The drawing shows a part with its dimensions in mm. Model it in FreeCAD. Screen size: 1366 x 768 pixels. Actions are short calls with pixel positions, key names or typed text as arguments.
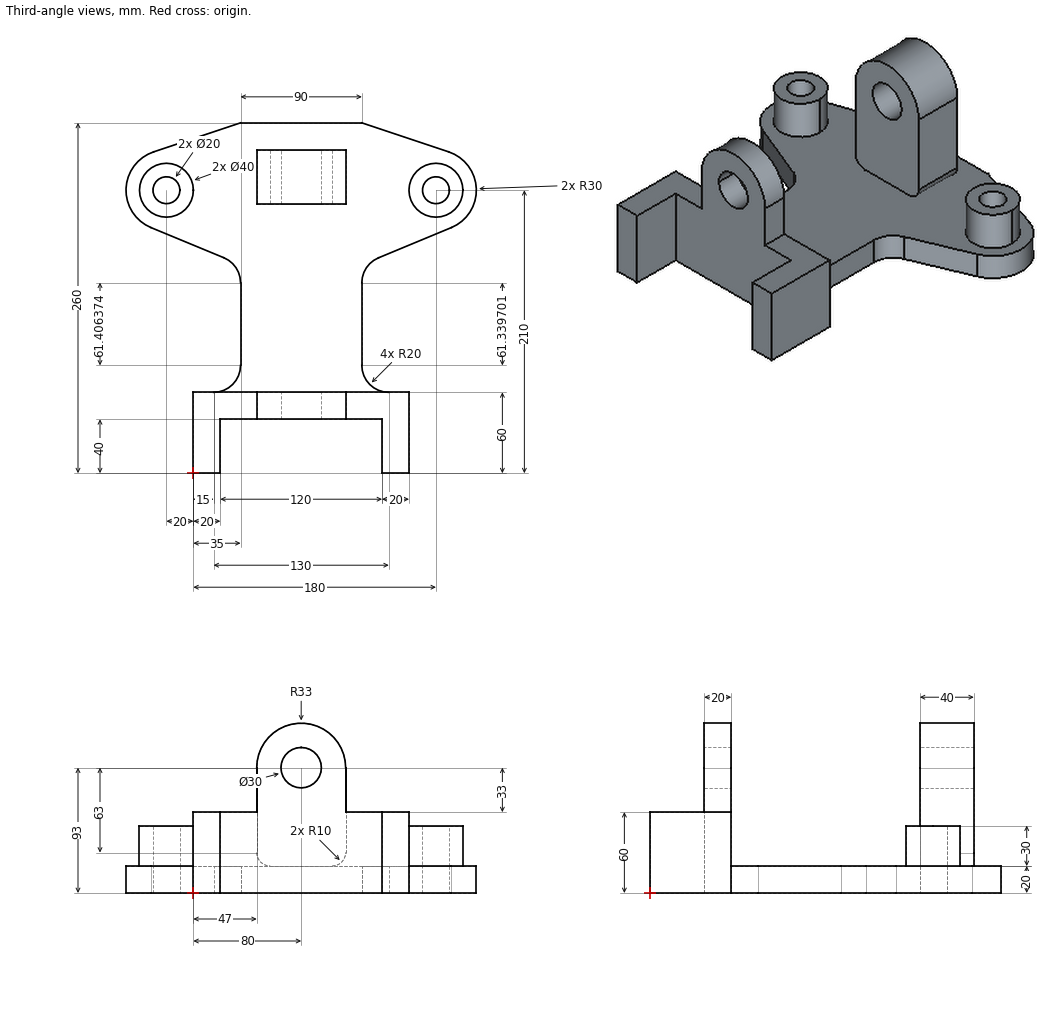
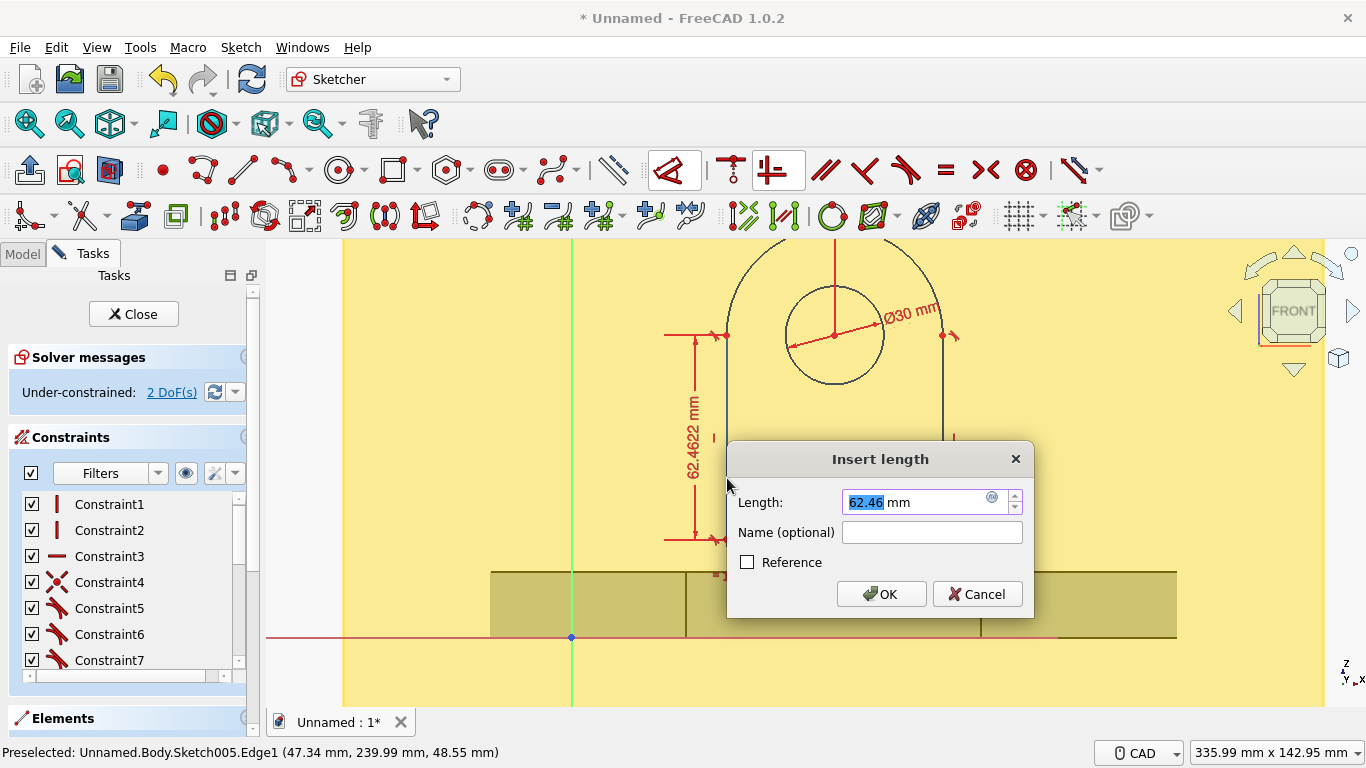
text(63)
key(Return)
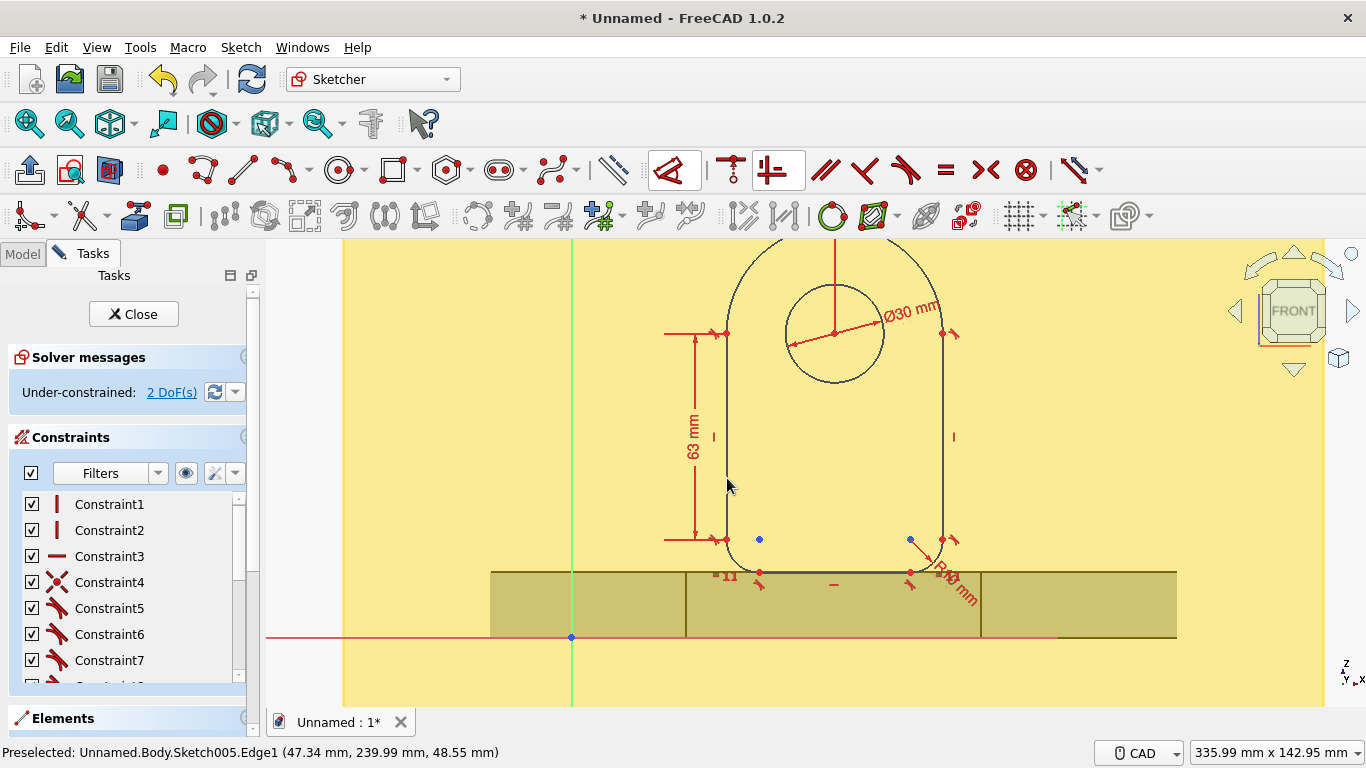
click(835, 334)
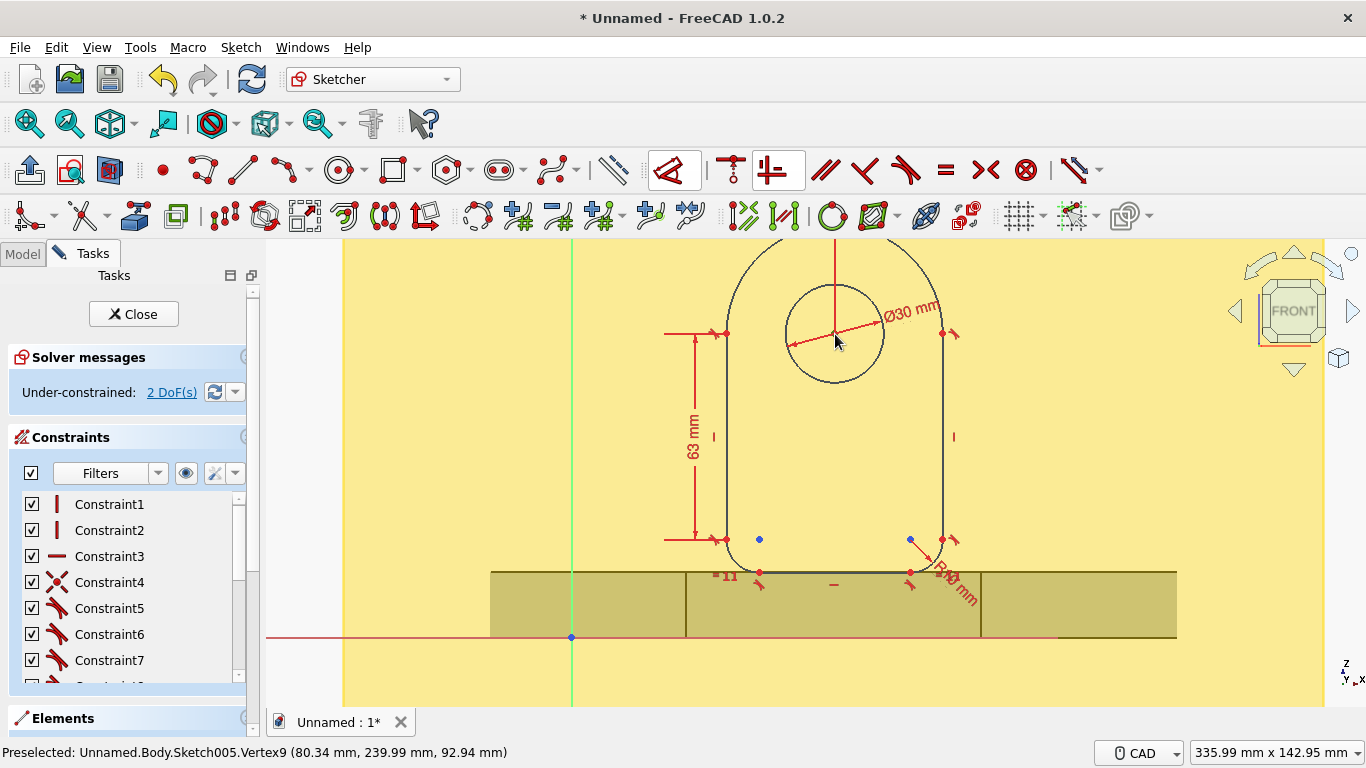
key(l)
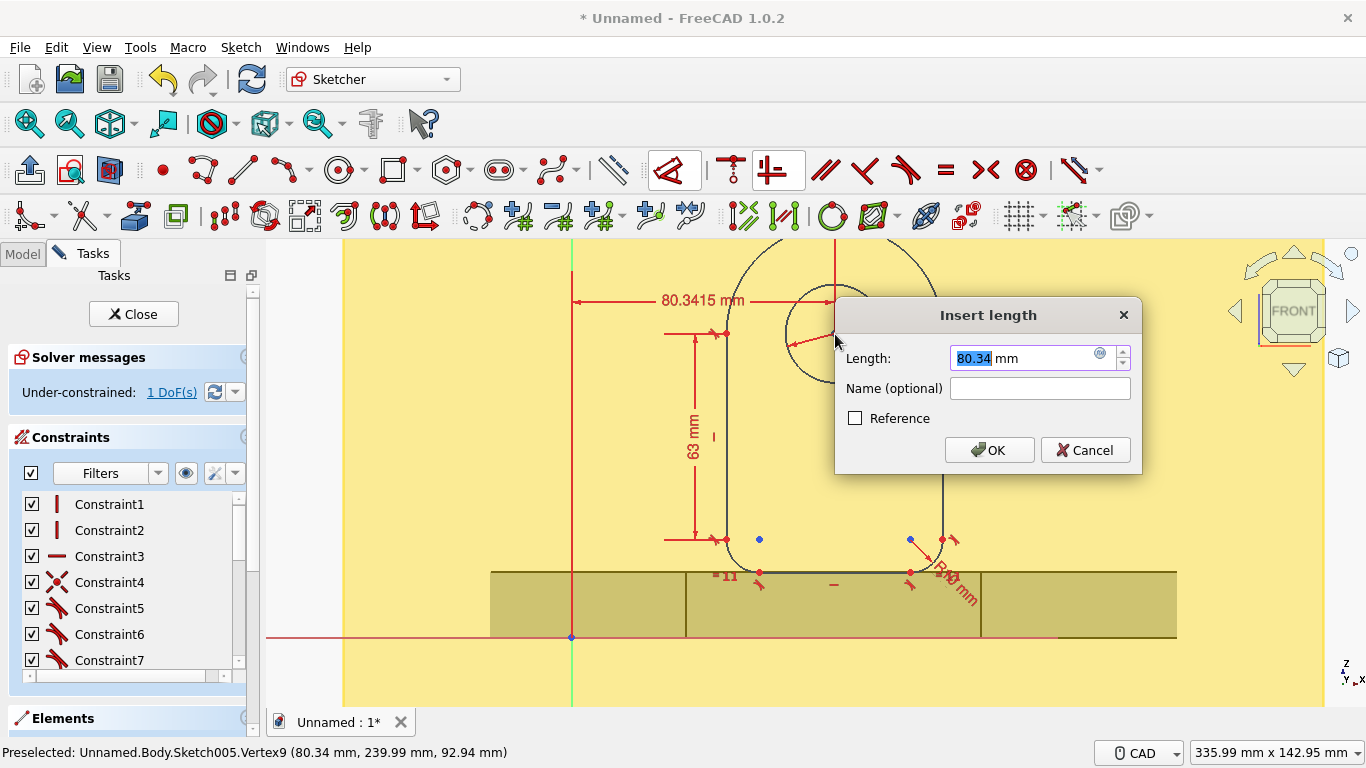
text(80)
key(Return)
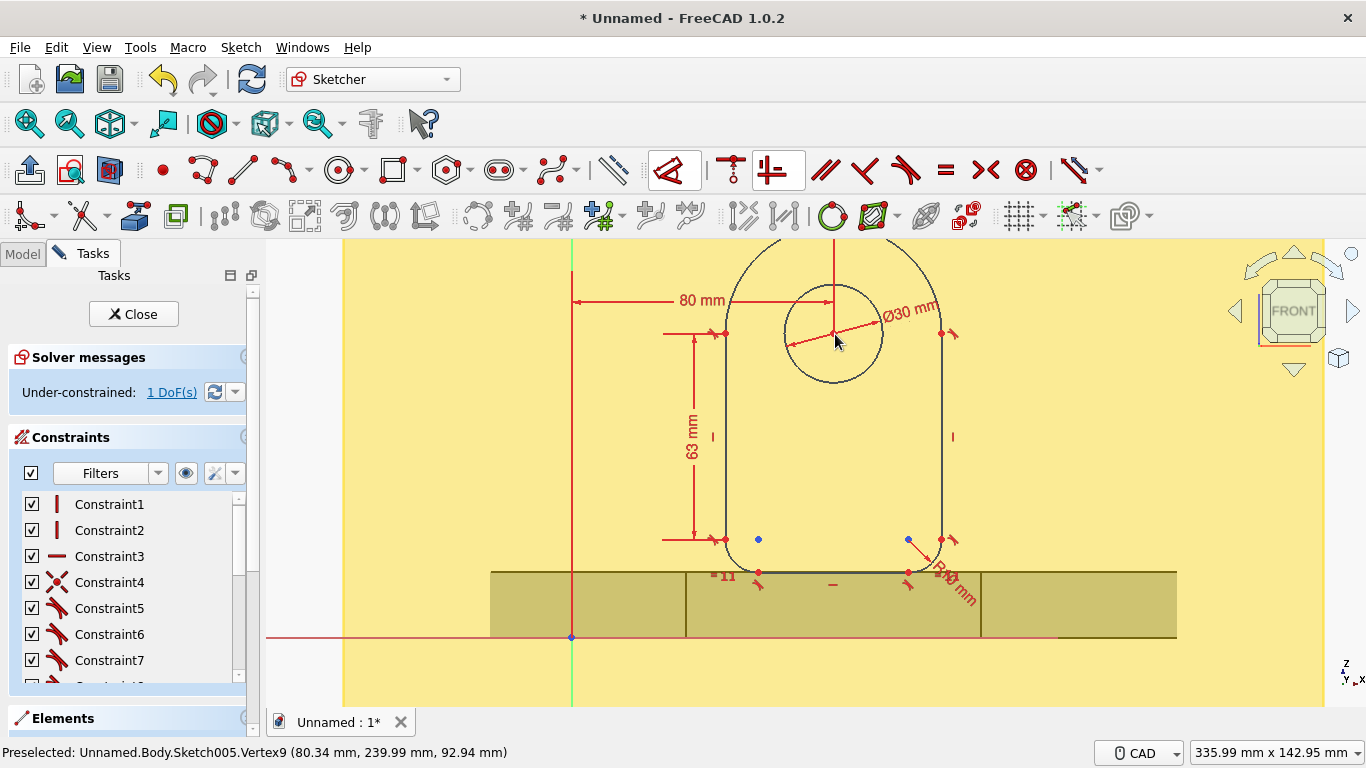
click(834, 334)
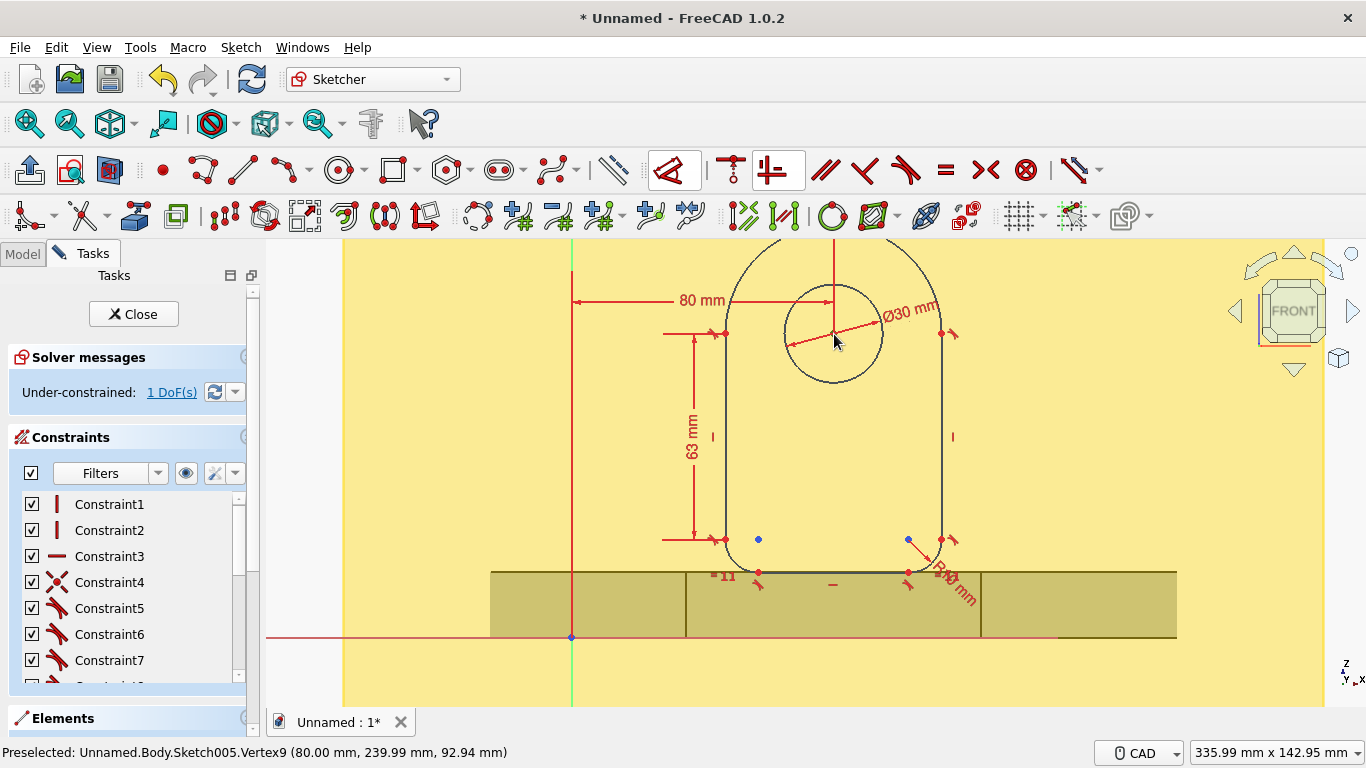
key(i)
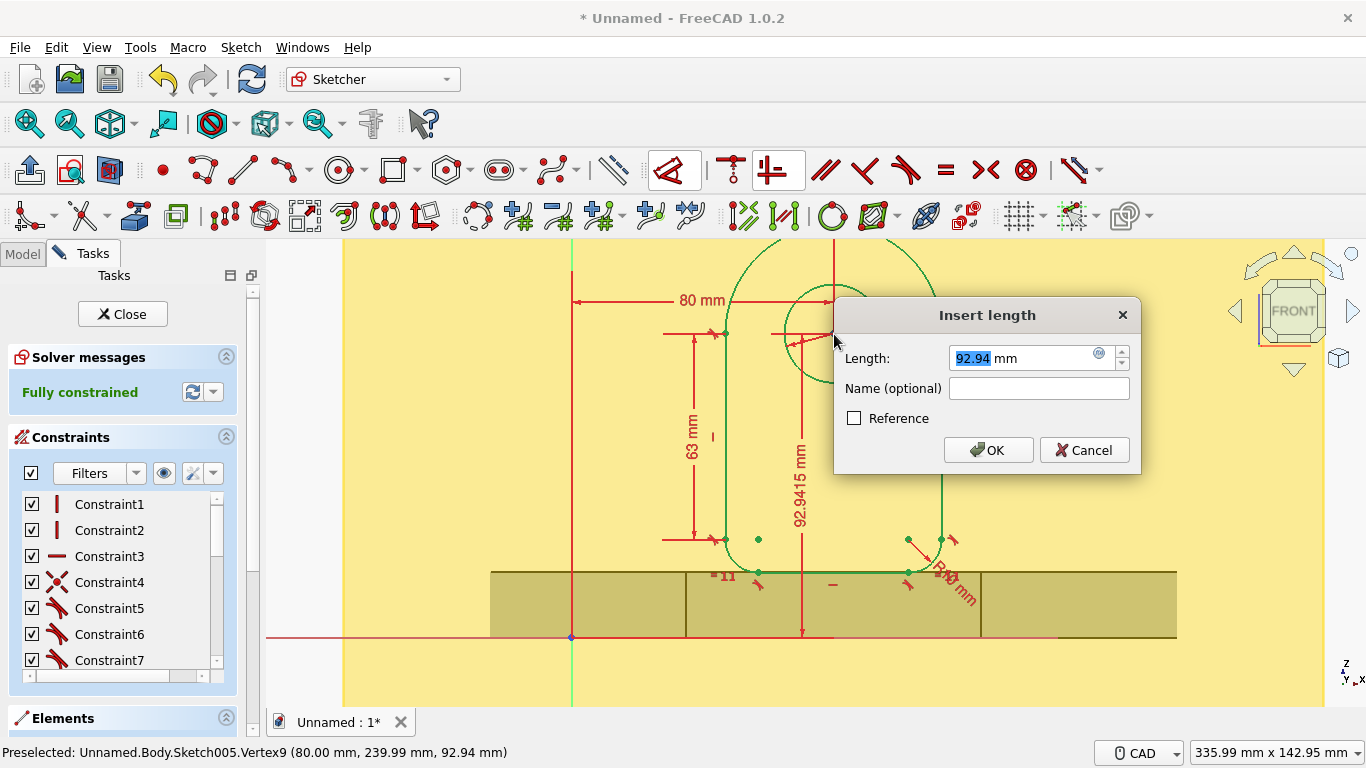
text(93)
key(Return)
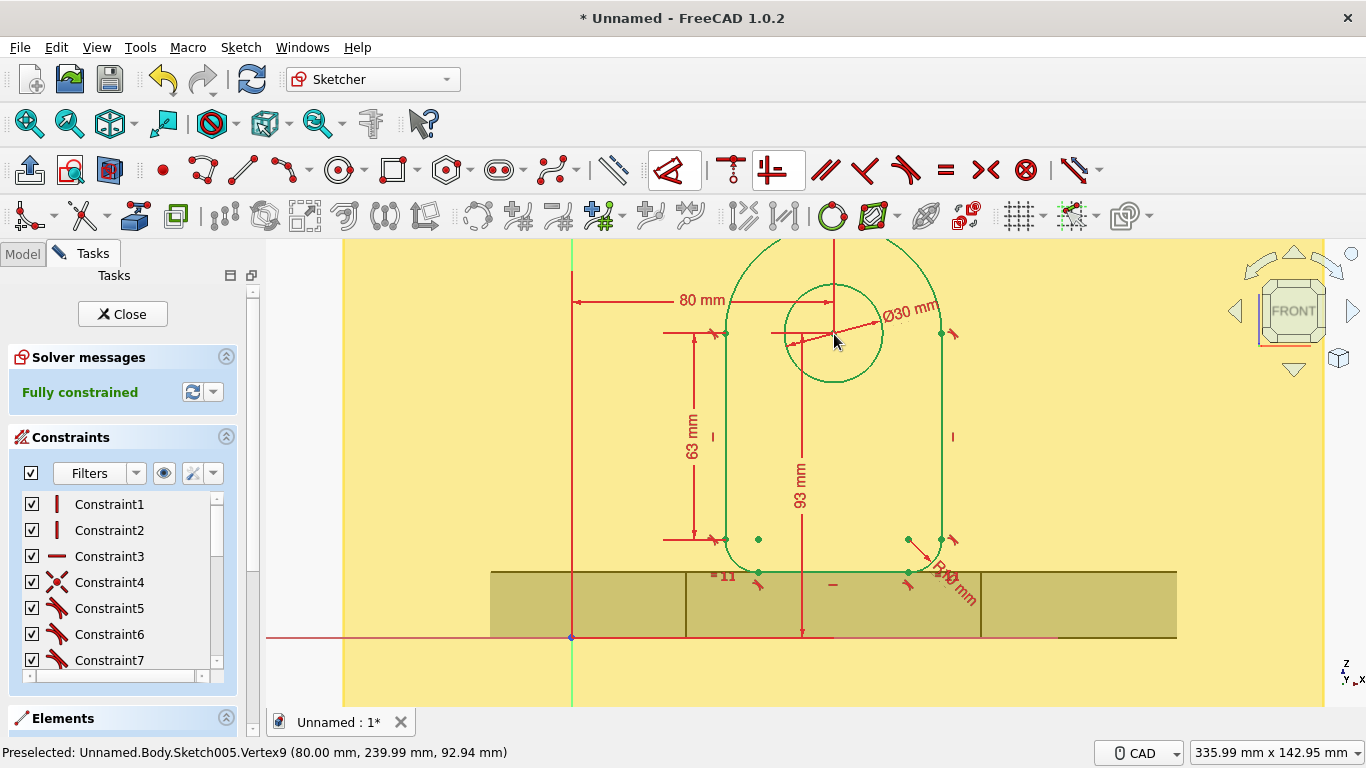
click(123, 314)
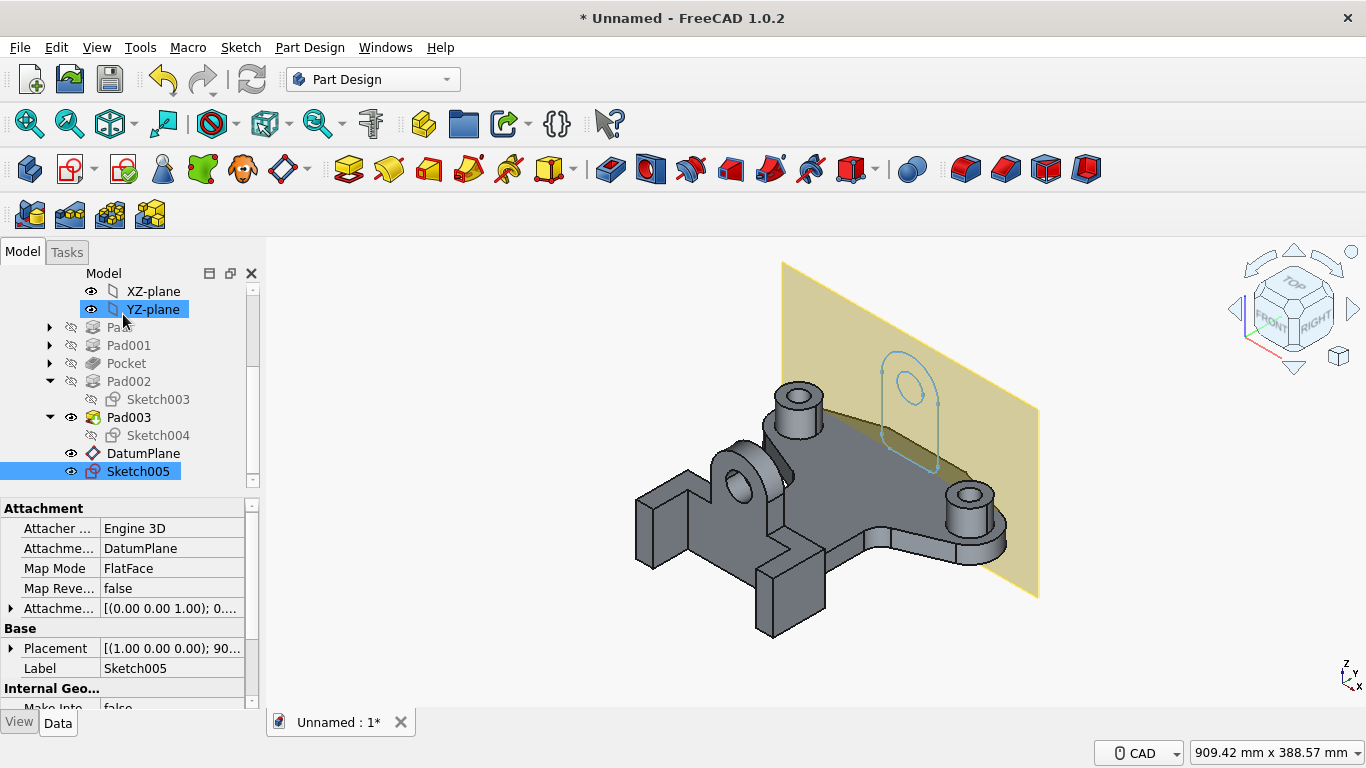
click(350, 170)